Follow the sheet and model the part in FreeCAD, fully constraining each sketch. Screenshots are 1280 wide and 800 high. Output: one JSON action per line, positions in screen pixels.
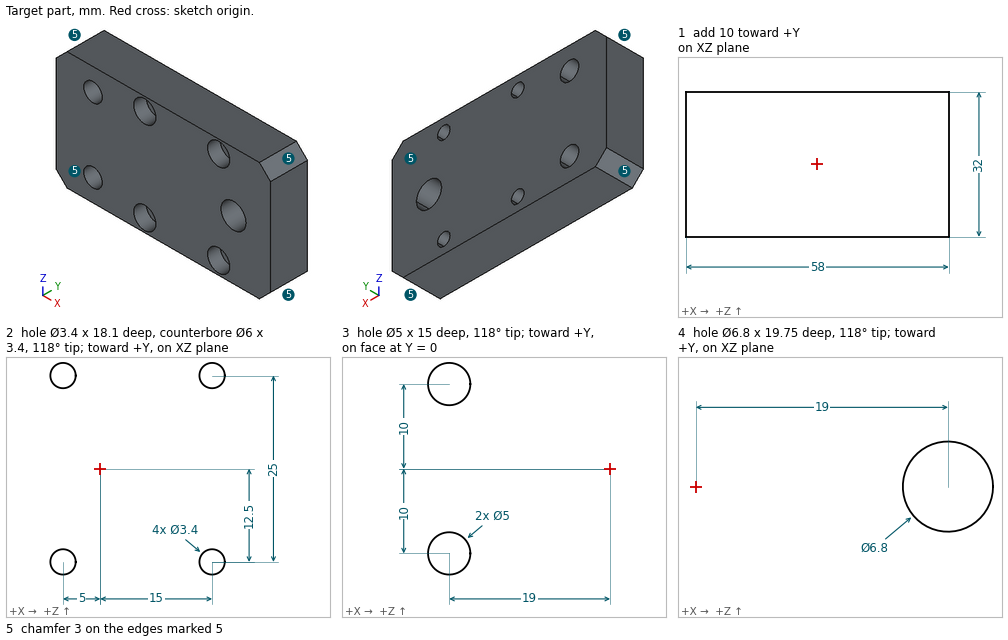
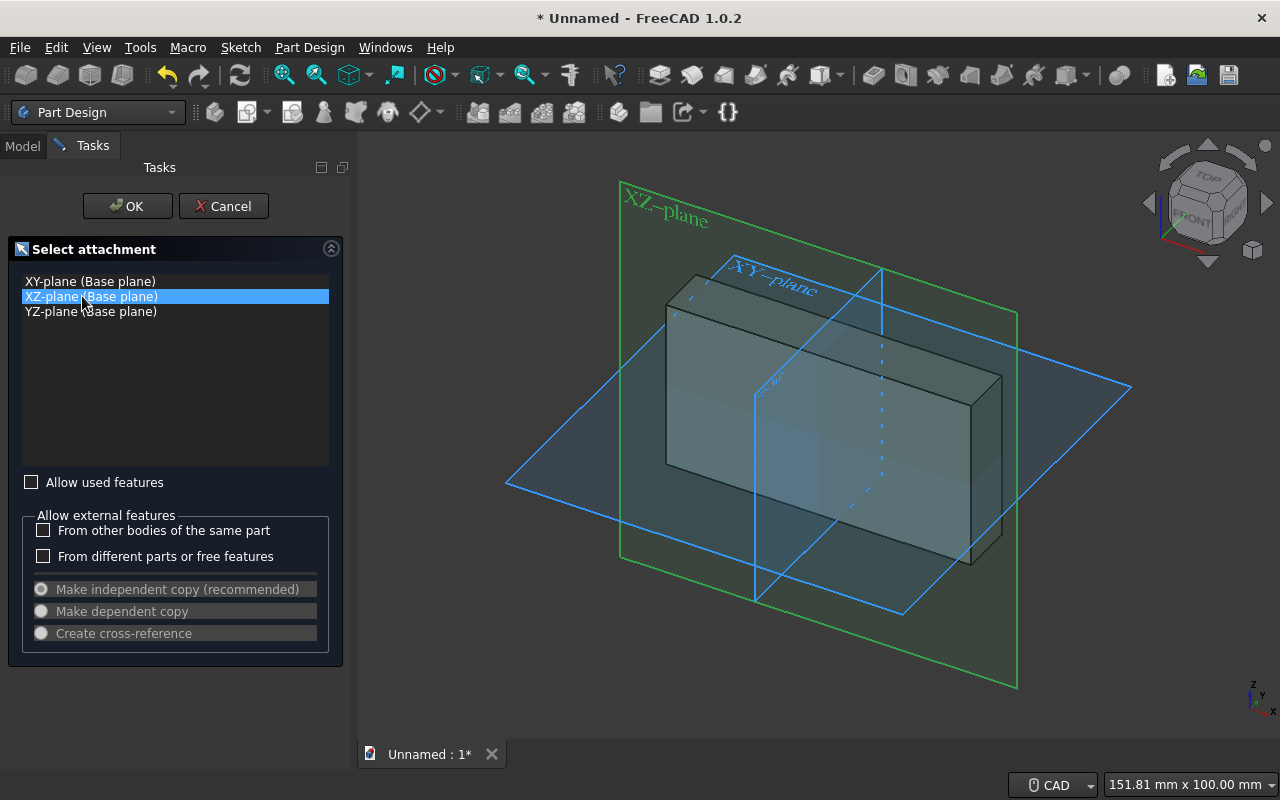
{"action": "left_click", "coordinate": [128, 206]}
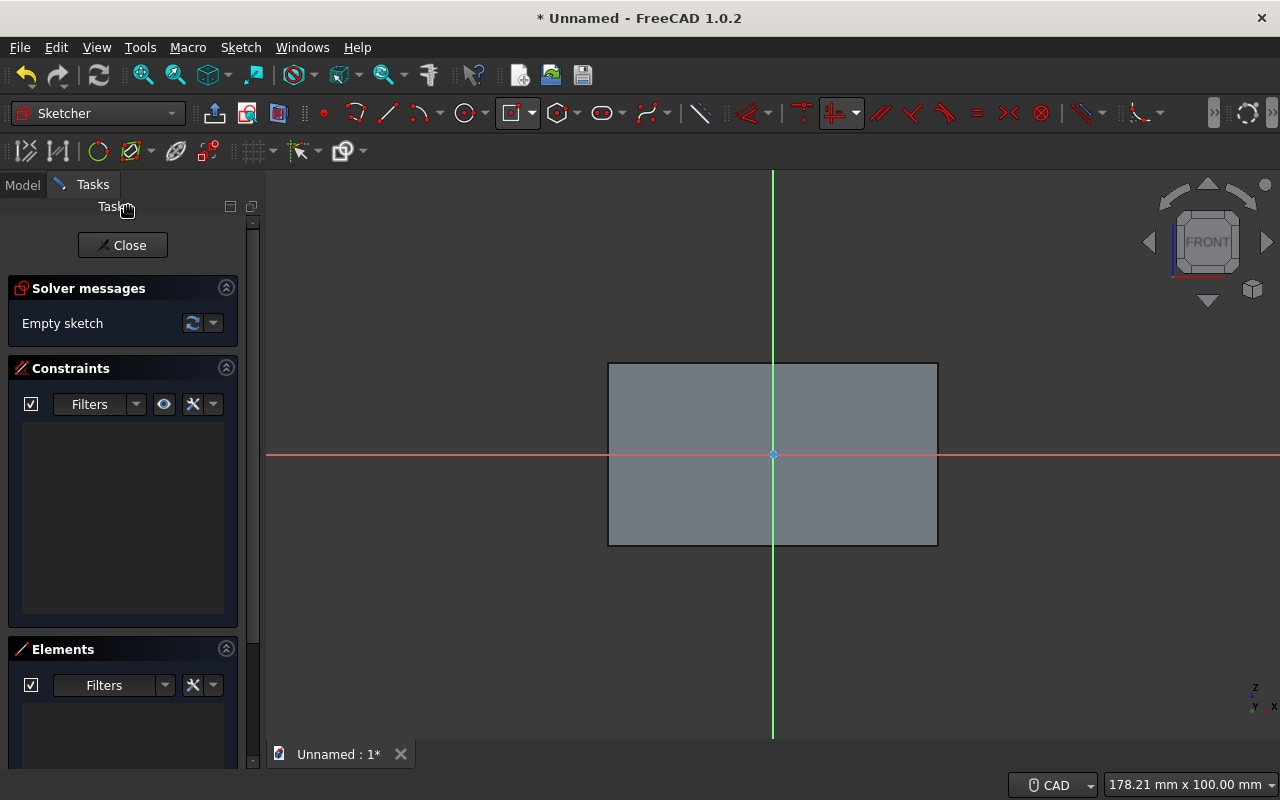
{"action": "scroll", "coordinate": [881, 455], "scroll_direction": "up", "scroll_amount": 4}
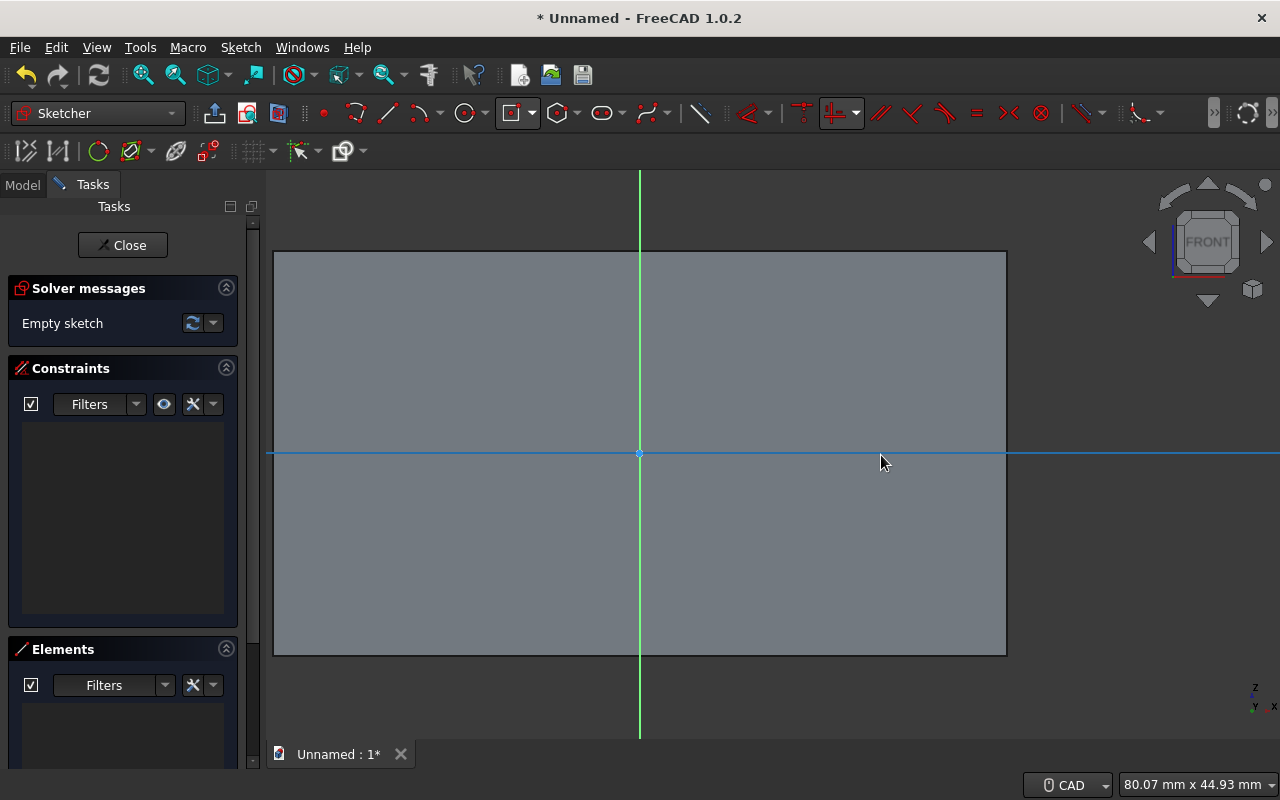
{"action": "left_click", "coordinate": [466, 114]}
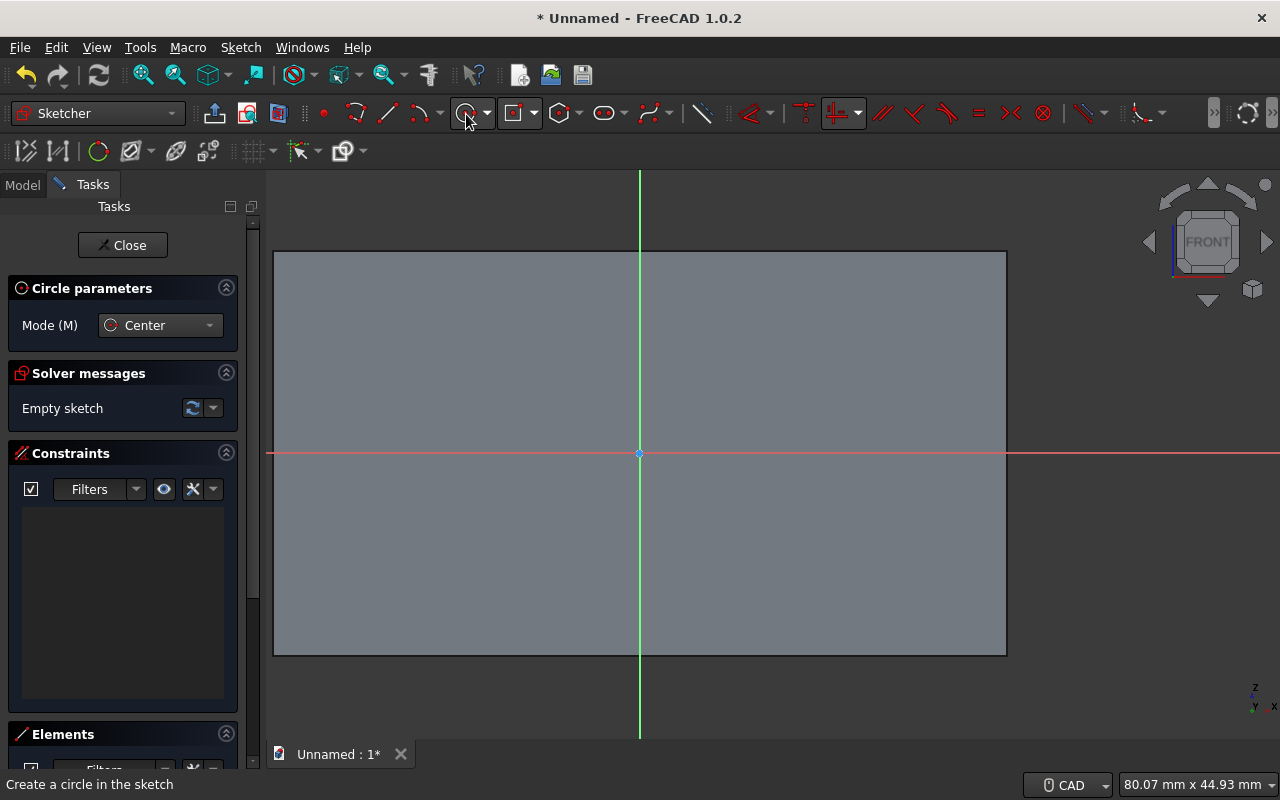
{"action": "left_click", "coordinate": [830, 612]}
{"action": "left_click", "coordinate": [845, 596]}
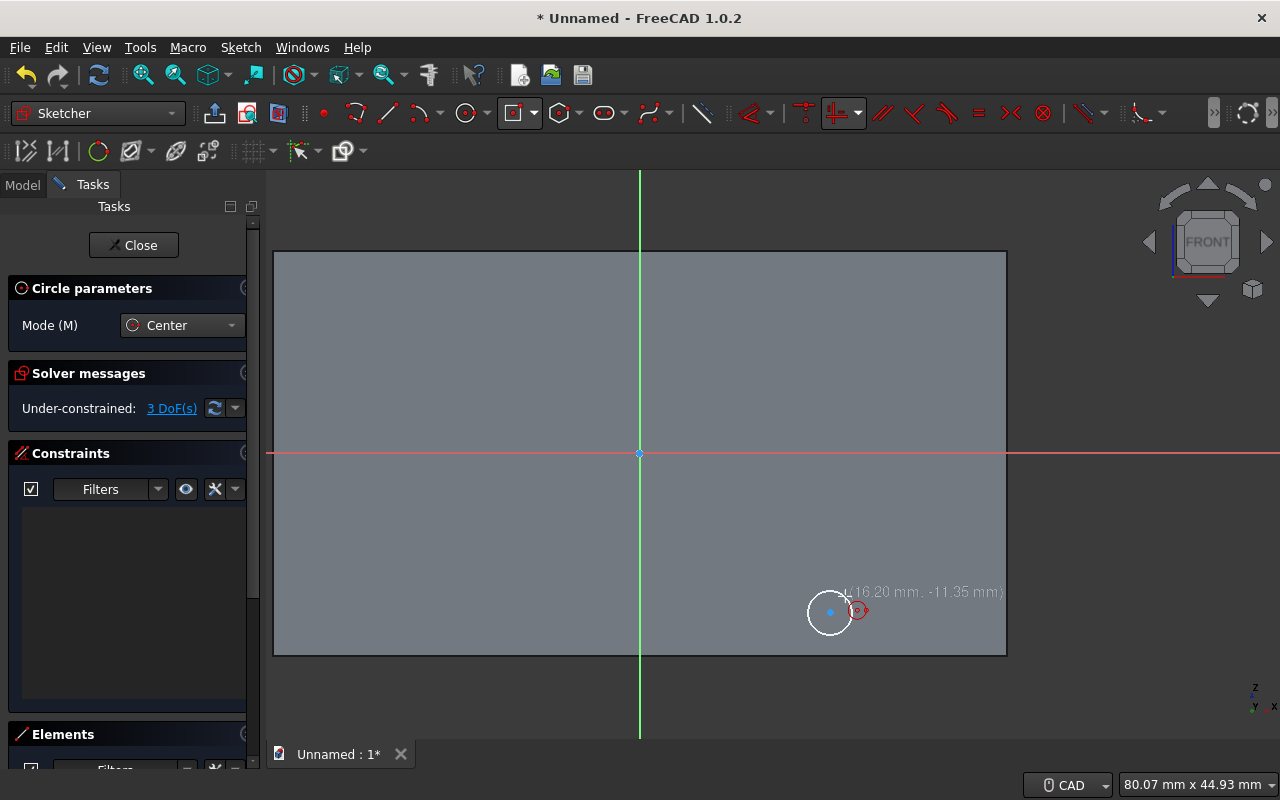
{"action": "left_click", "coordinate": [577, 612]}
{"action": "left_click", "coordinate": [592, 596]}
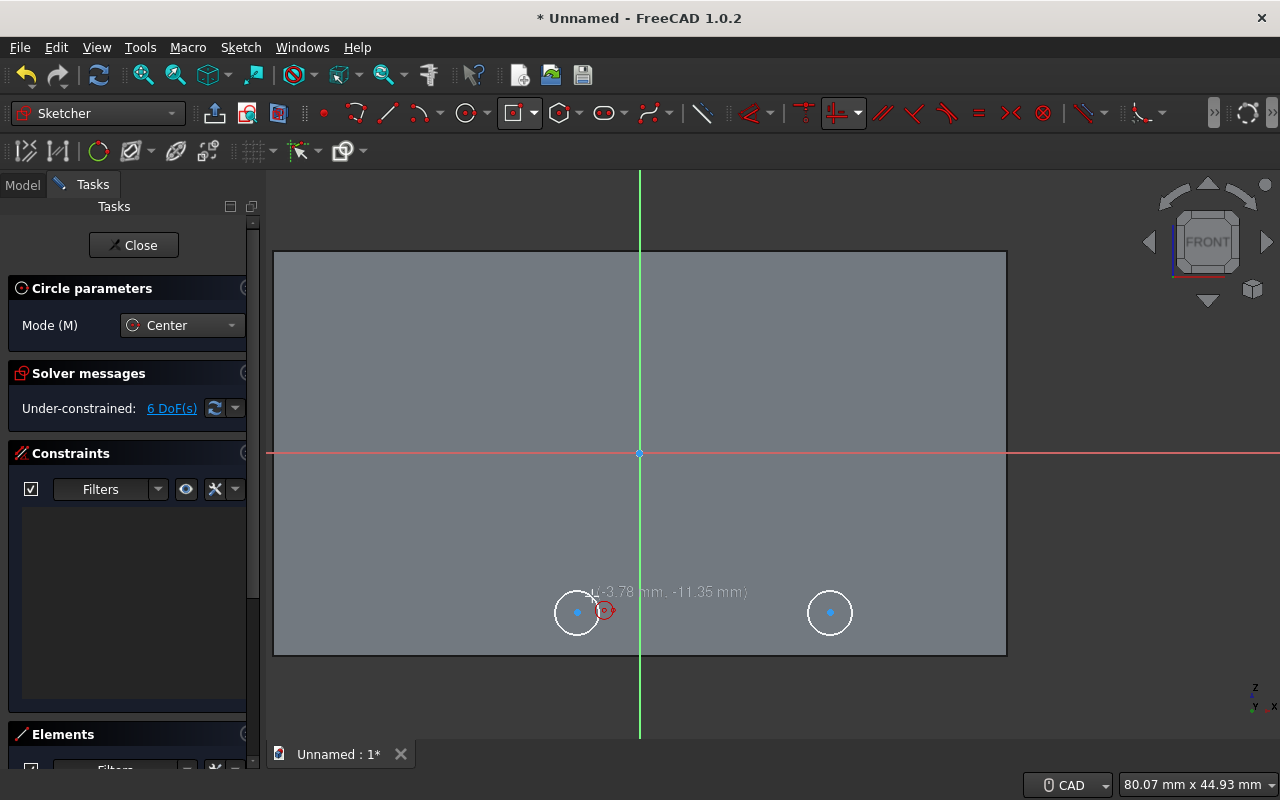
{"action": "left_click", "coordinate": [830, 295]}
{"action": "left_click", "coordinate": [845, 280]}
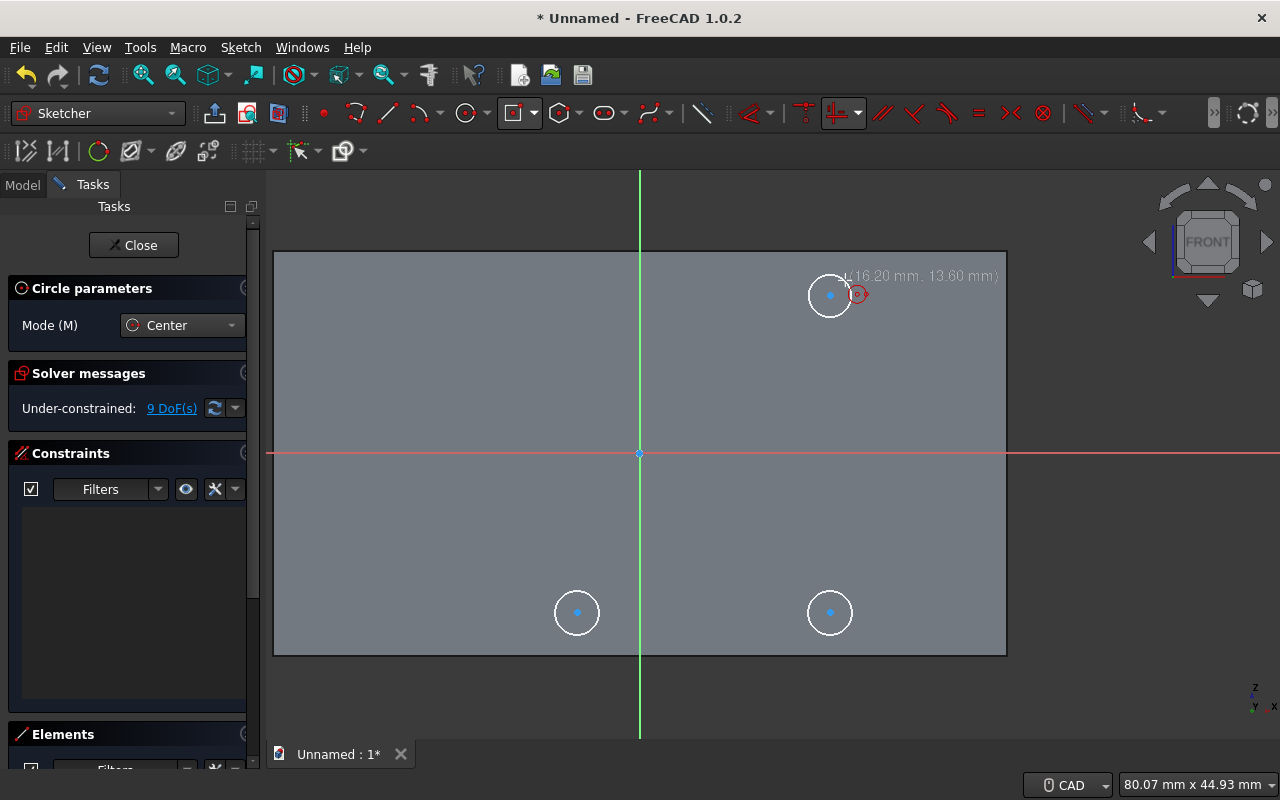
{"action": "left_click", "coordinate": [577, 295]}
{"action": "left_click", "coordinate": [592, 280]}
{"action": "key", "text": "Escape"}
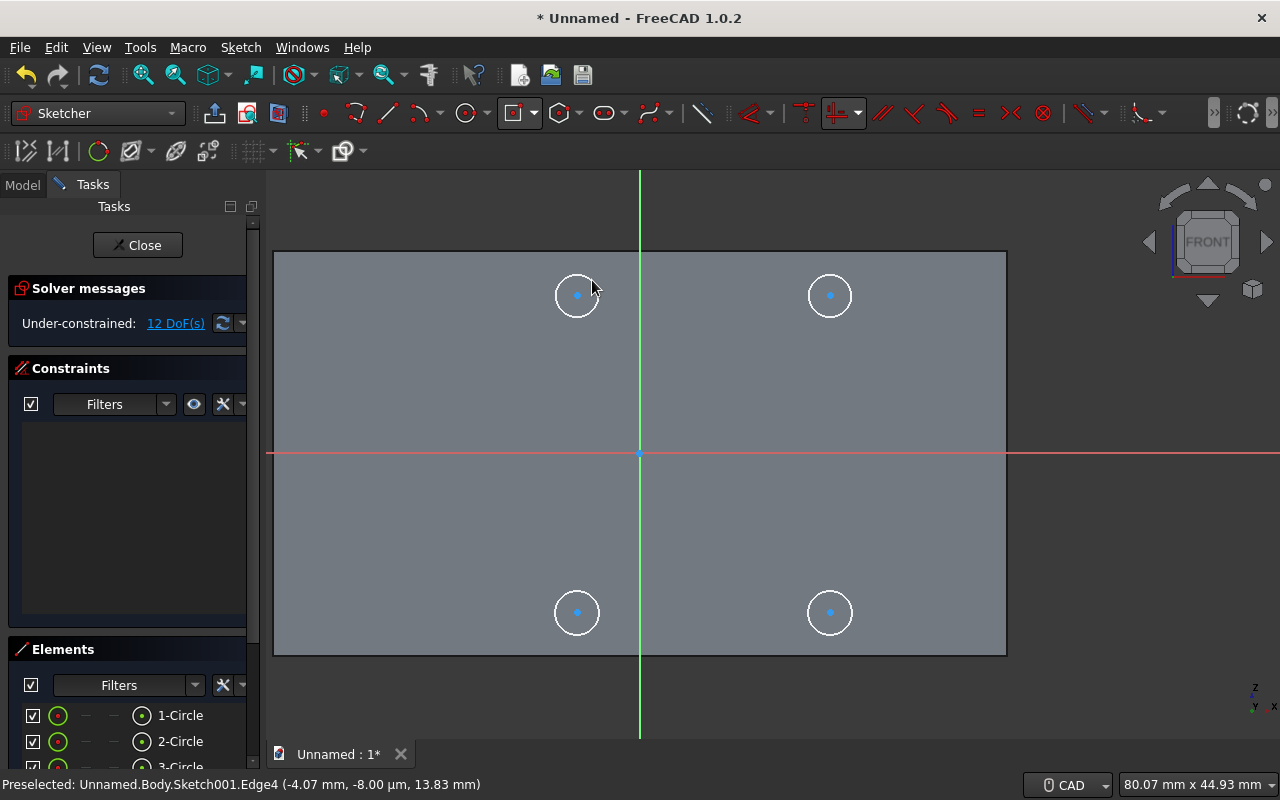
{"action": "left_click", "coordinate": [845, 597]}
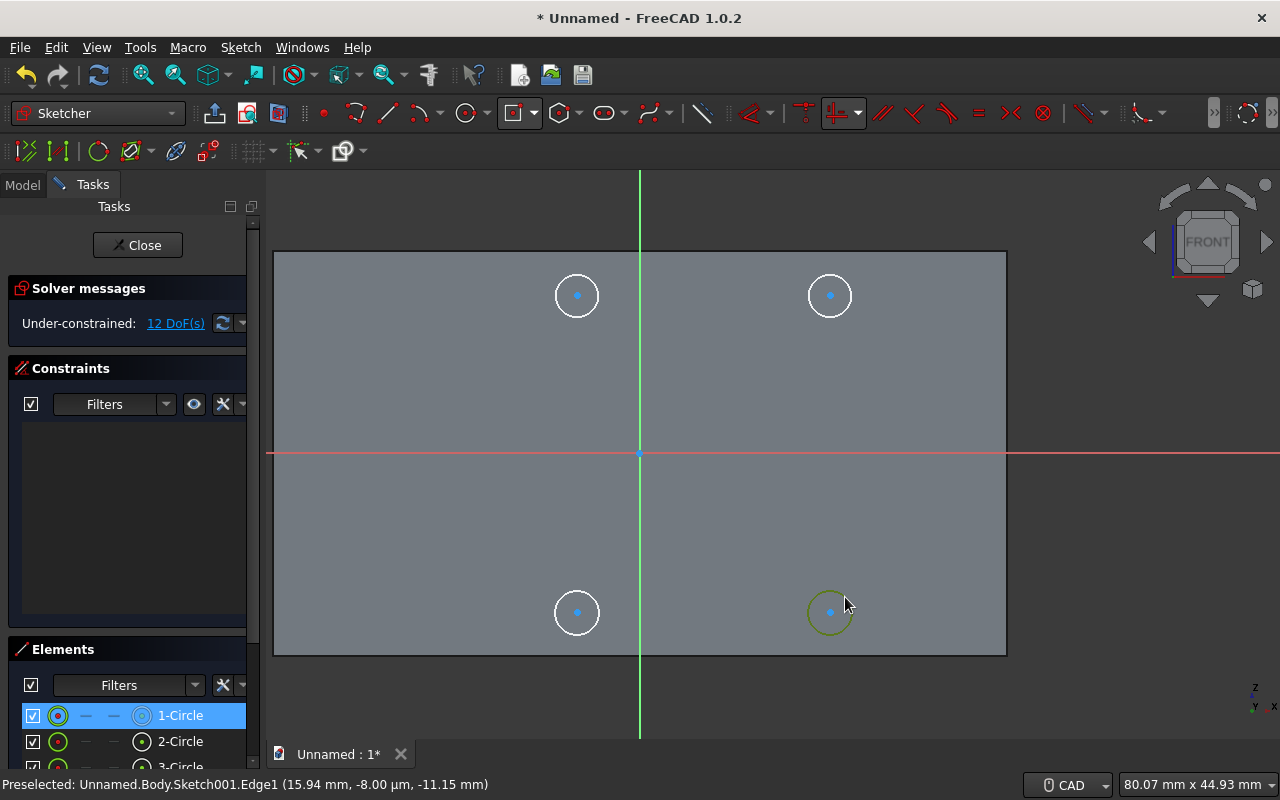
{"action": "left_click", "coordinate": [592, 597]}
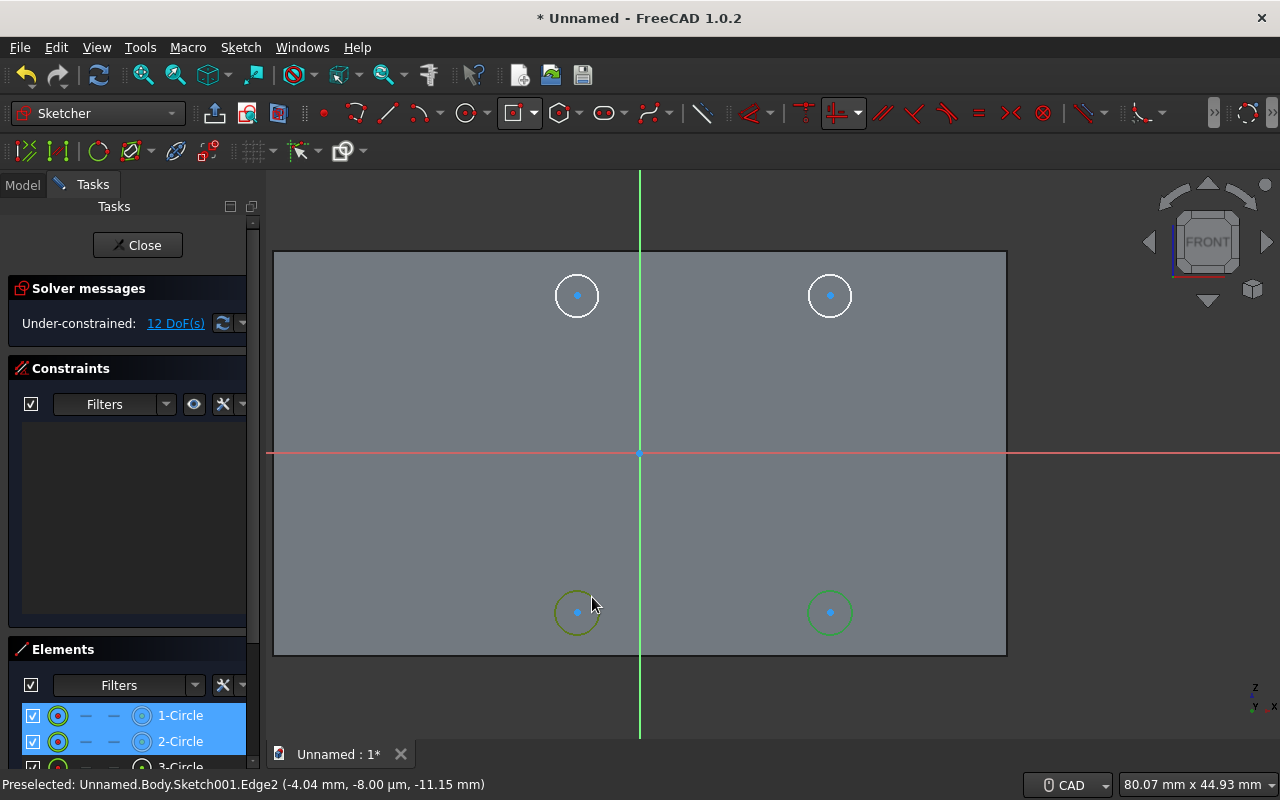
{"action": "left_click", "coordinate": [845, 281]}